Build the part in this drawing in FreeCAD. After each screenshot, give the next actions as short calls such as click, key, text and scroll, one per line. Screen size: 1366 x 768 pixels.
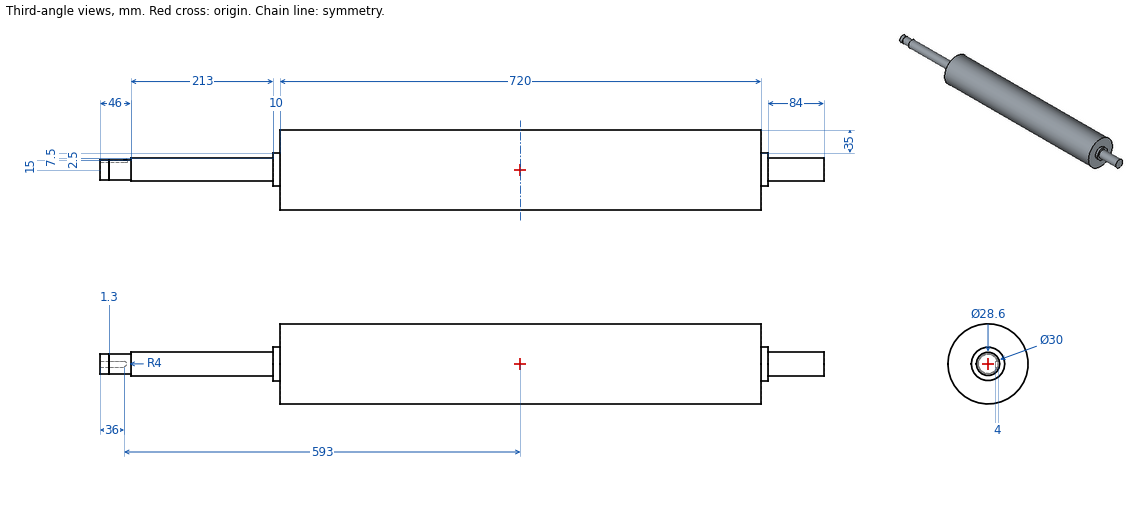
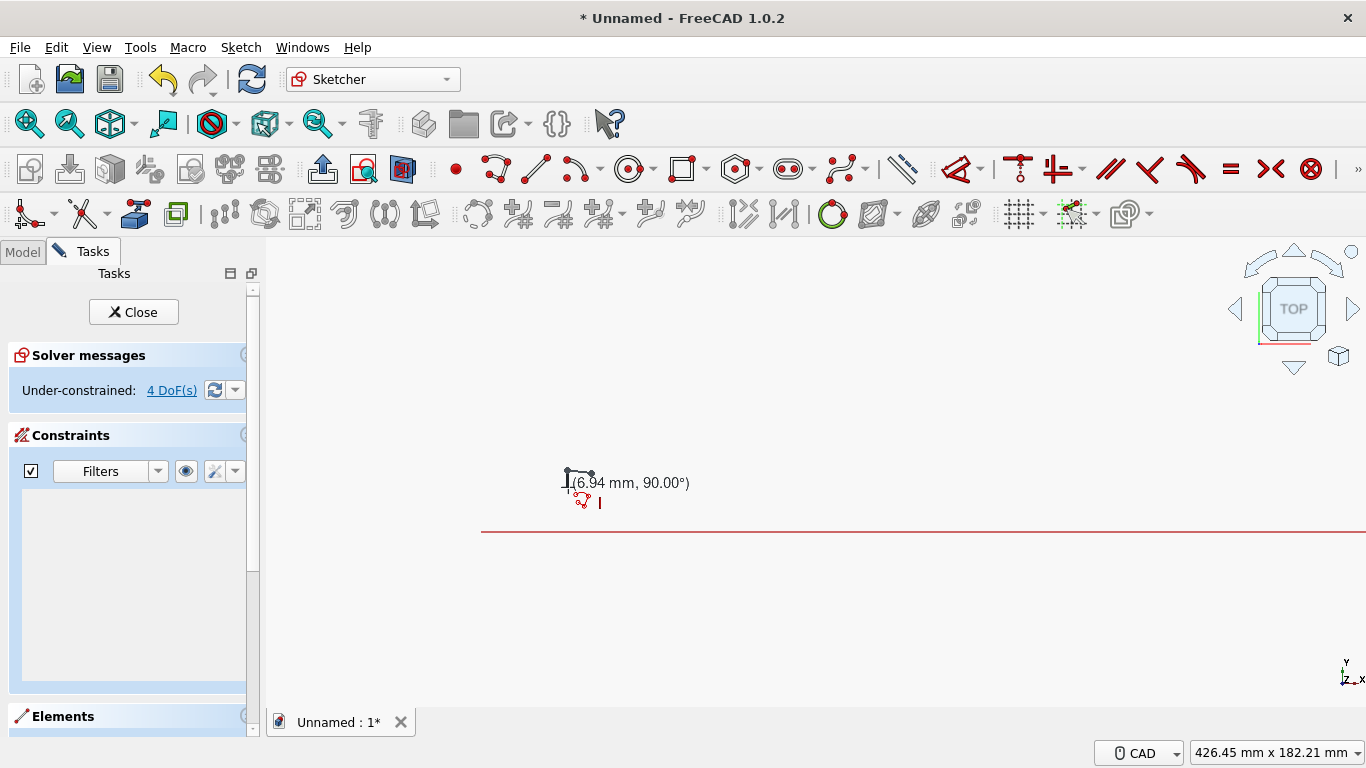
click(568, 487)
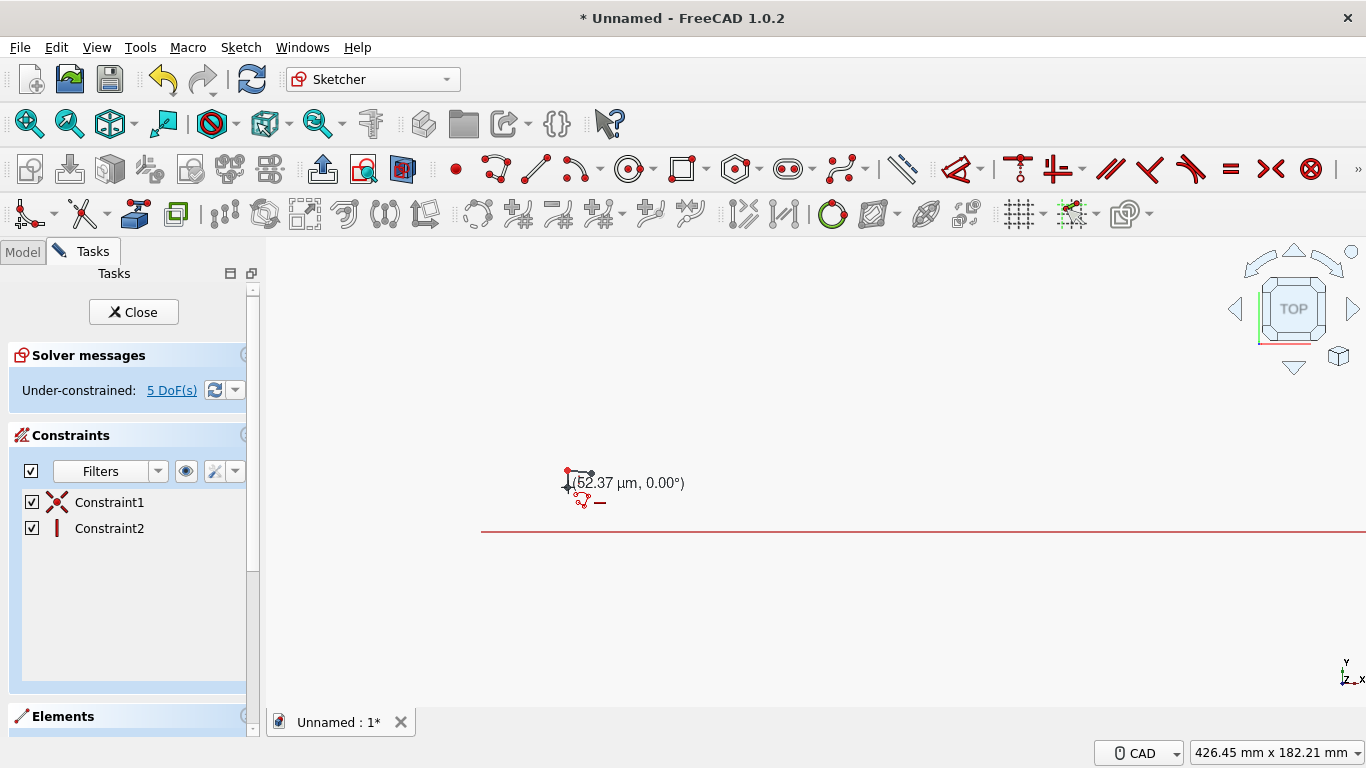
scroll(568, 478, down, 7)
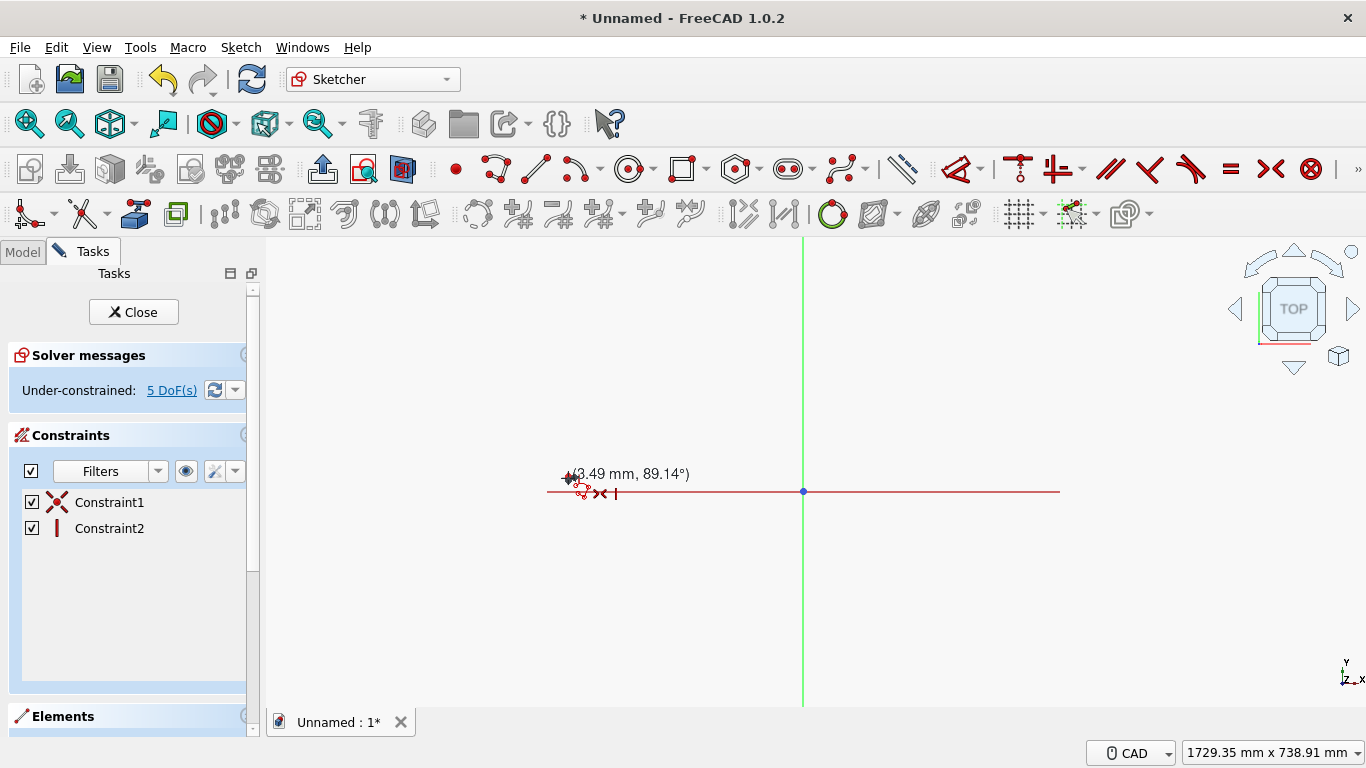
scroll(433, 481, up, 2)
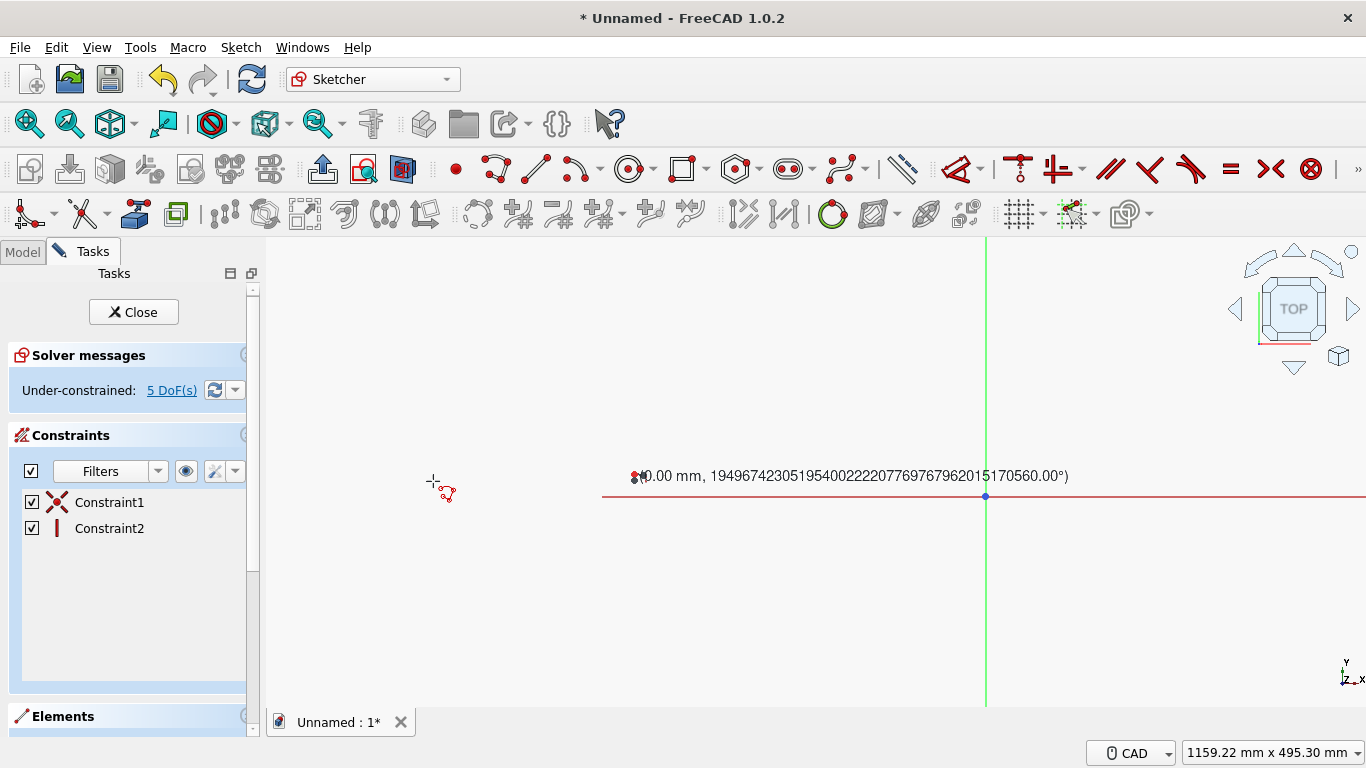
click(432, 480)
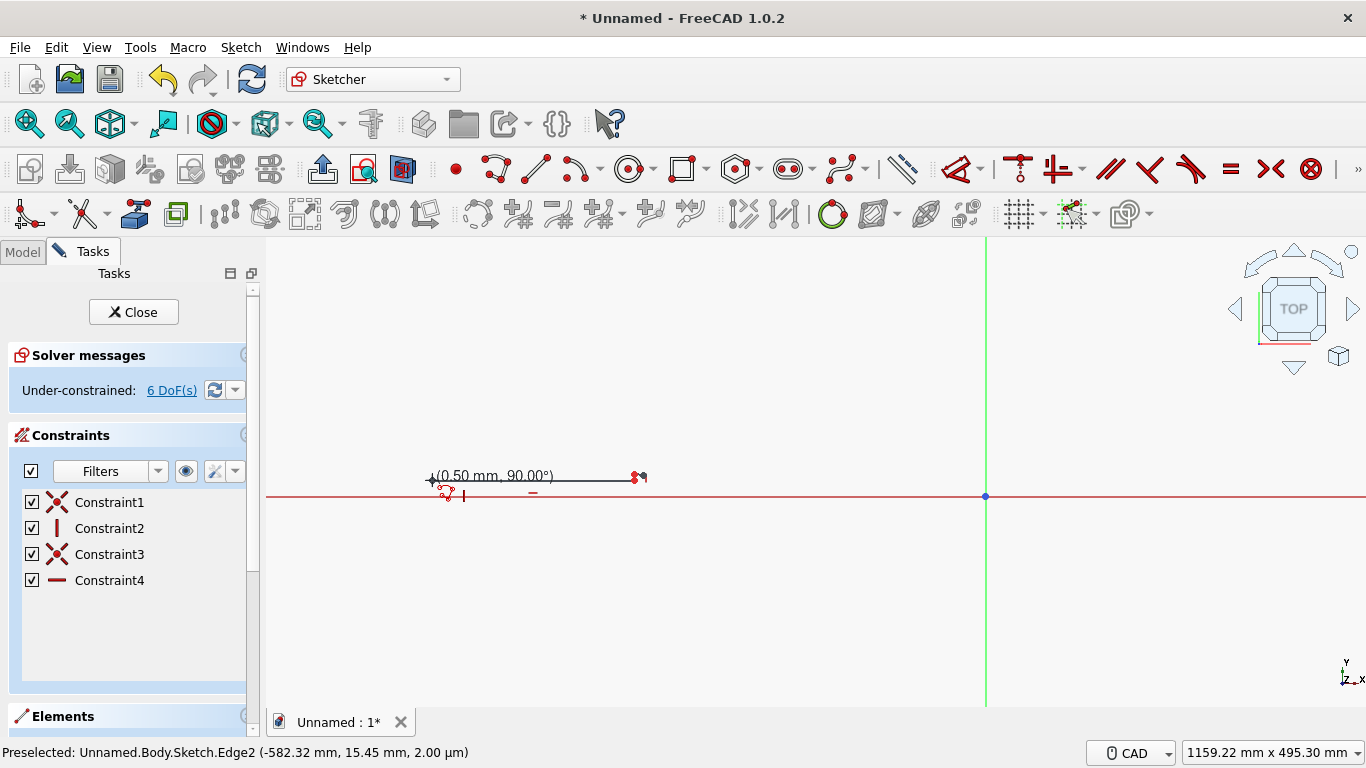
scroll(432, 482, up, 10)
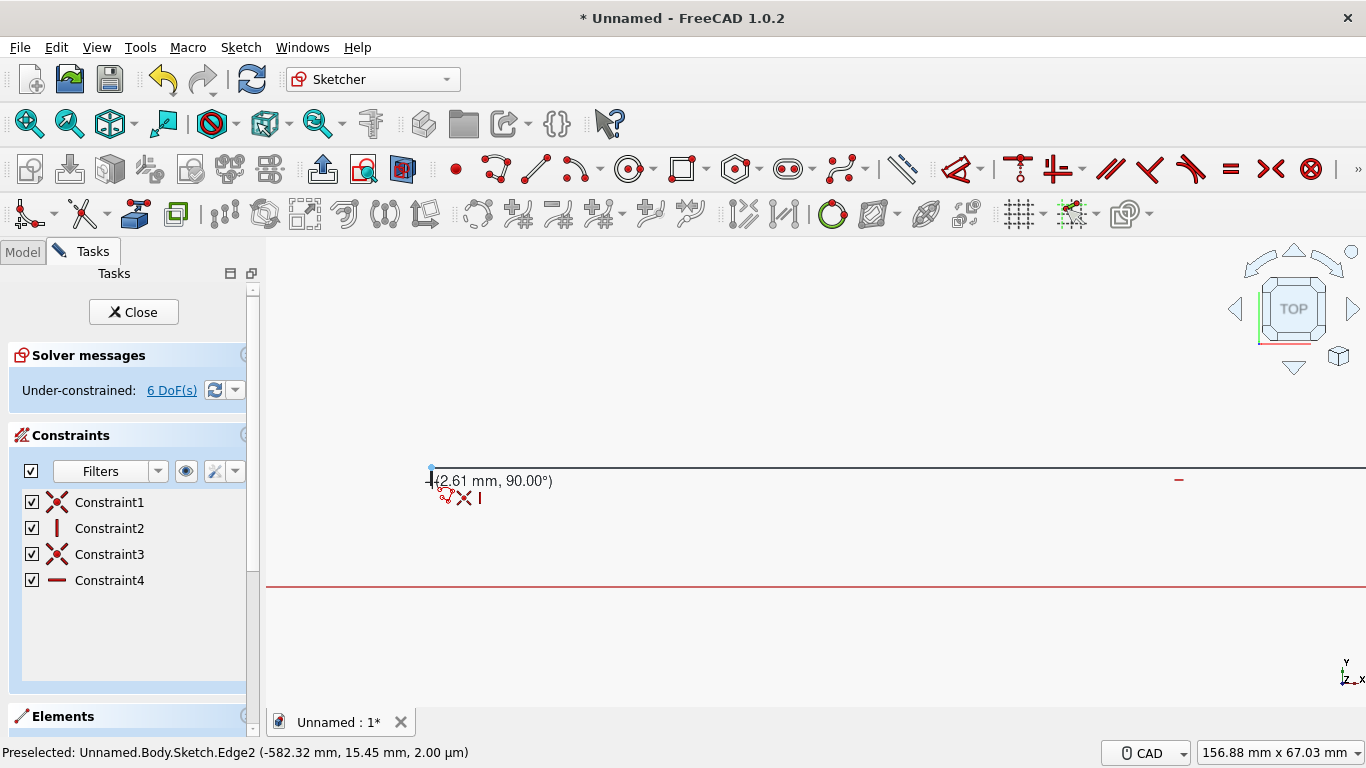
click(431, 482)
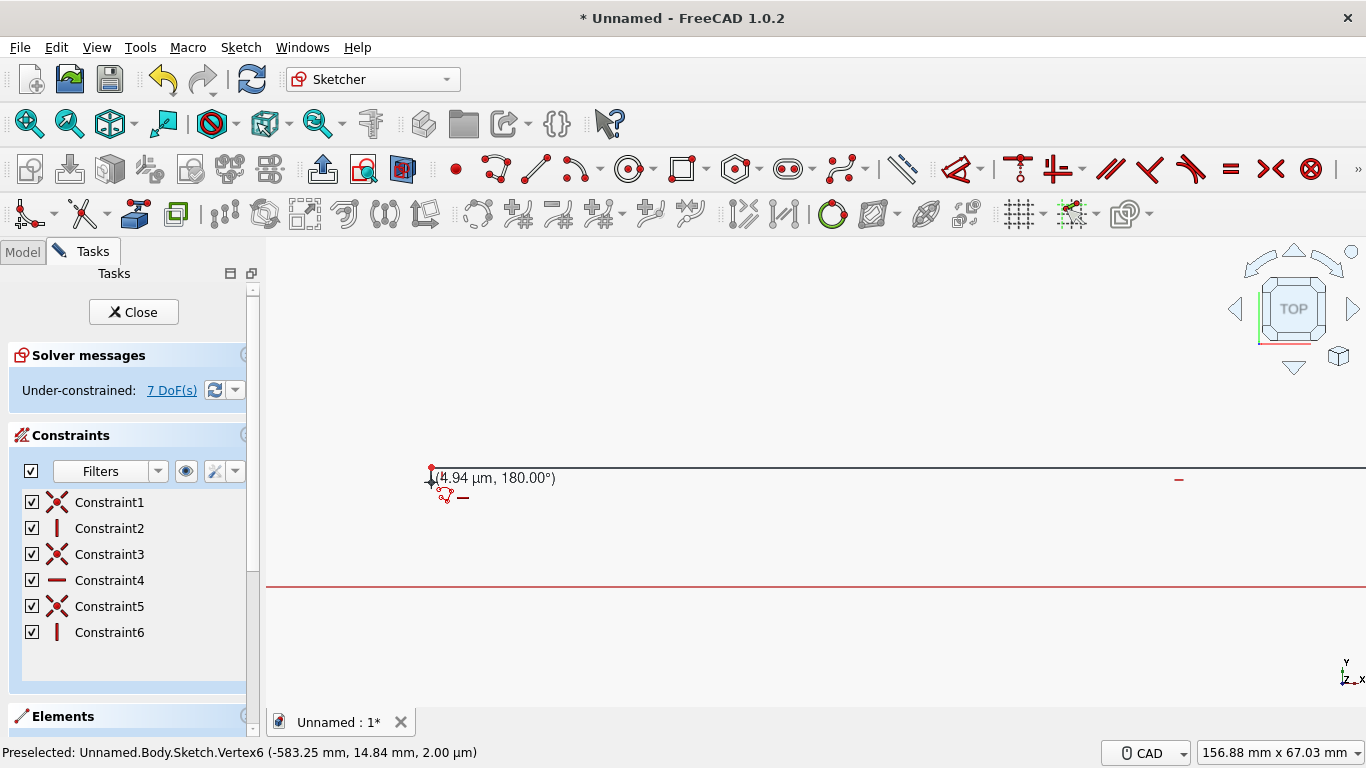
scroll(432, 482, down, 12)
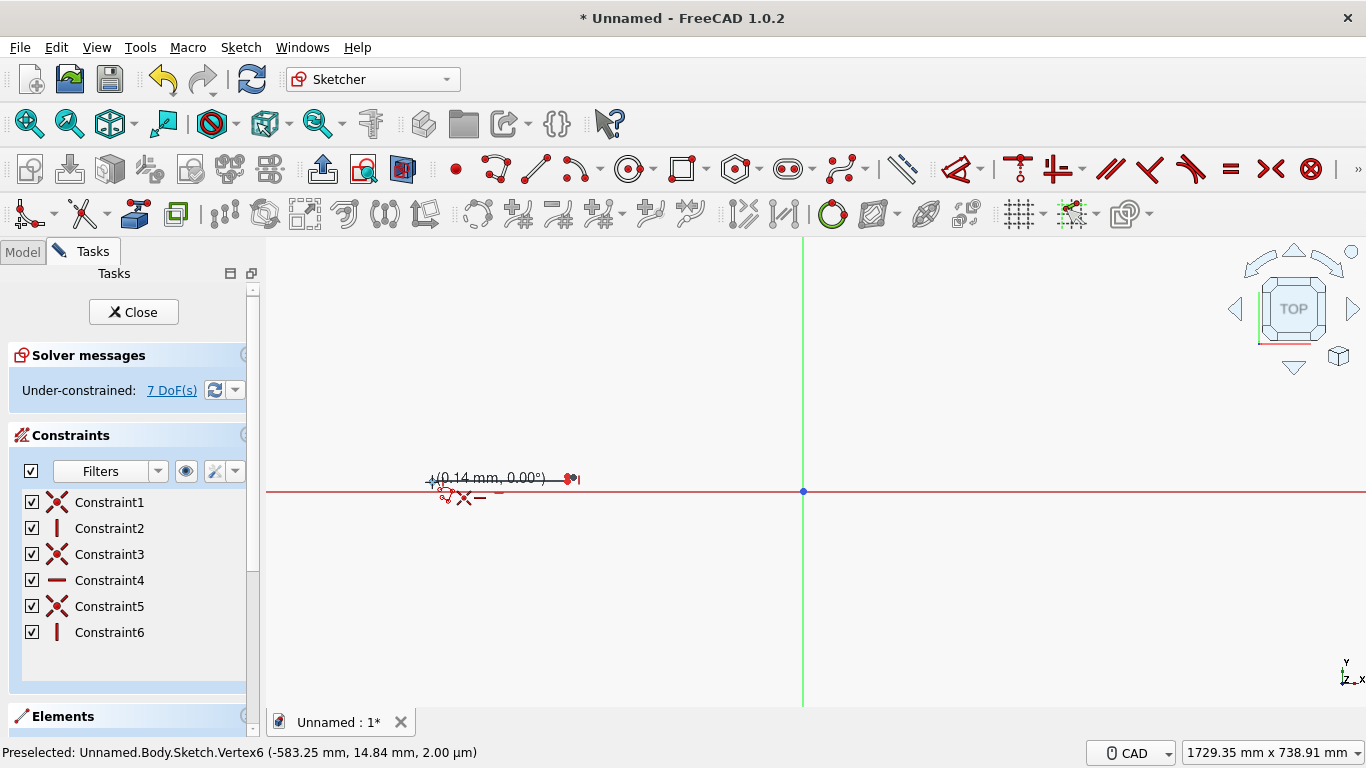
scroll(403, 482, up, 3)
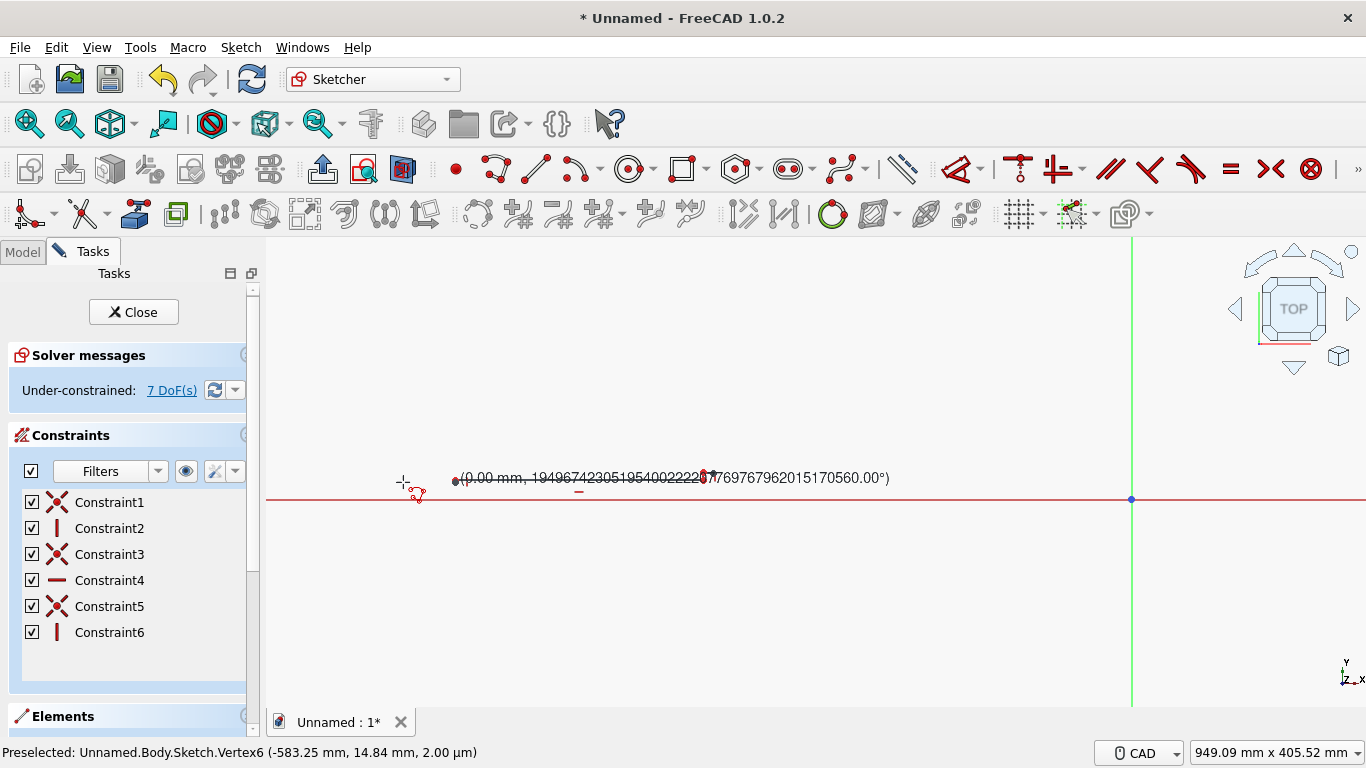
click(403, 482)
click(403, 500)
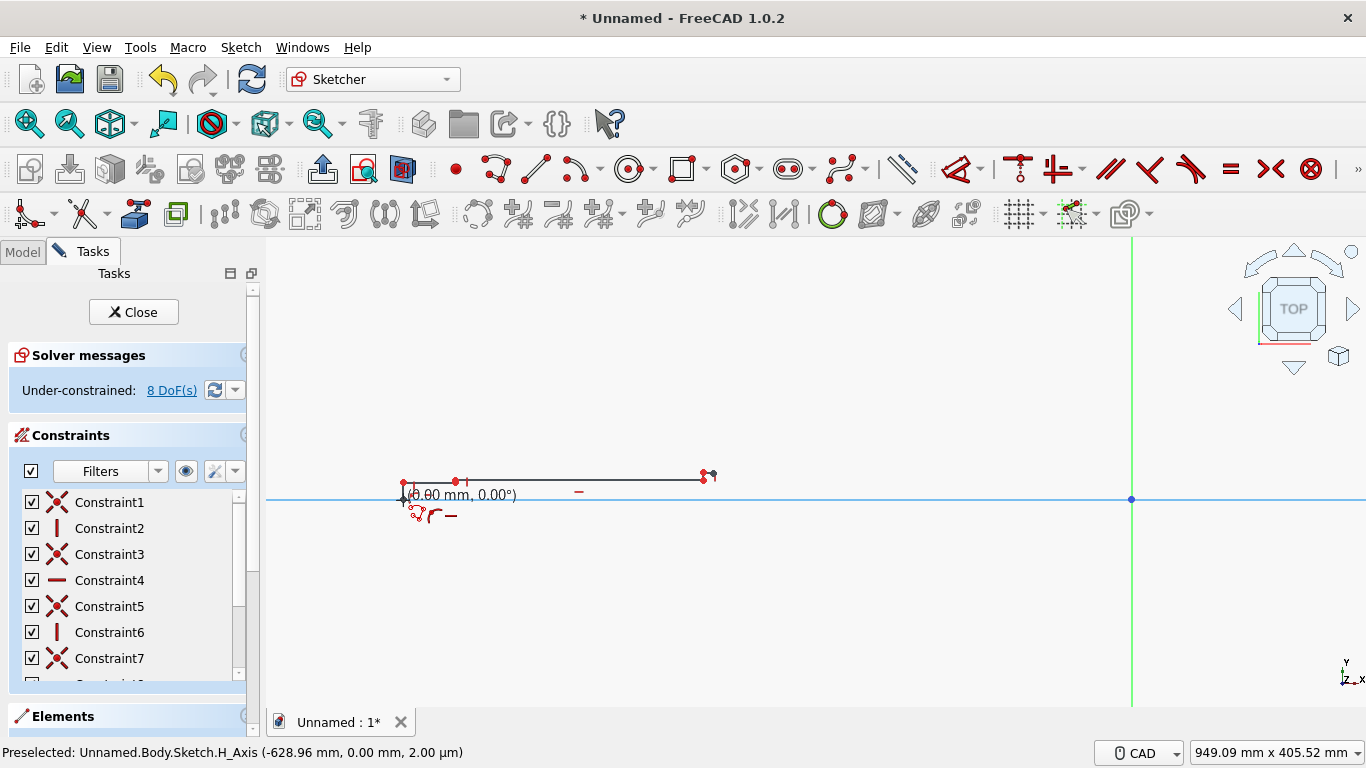
scroll(403, 480, down, 3)